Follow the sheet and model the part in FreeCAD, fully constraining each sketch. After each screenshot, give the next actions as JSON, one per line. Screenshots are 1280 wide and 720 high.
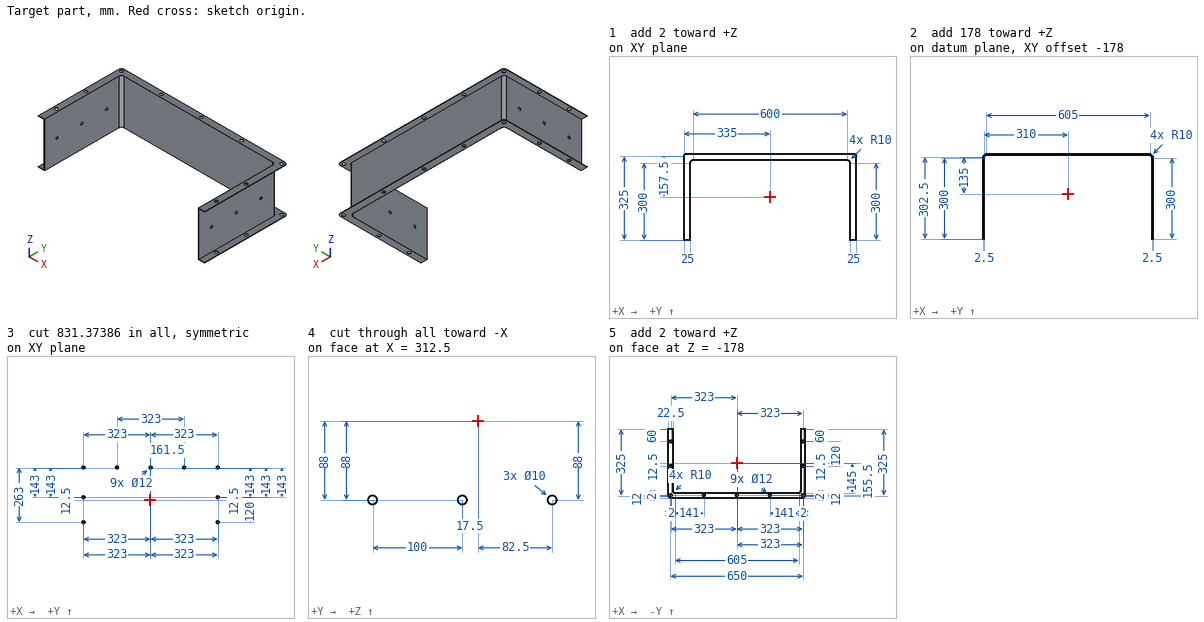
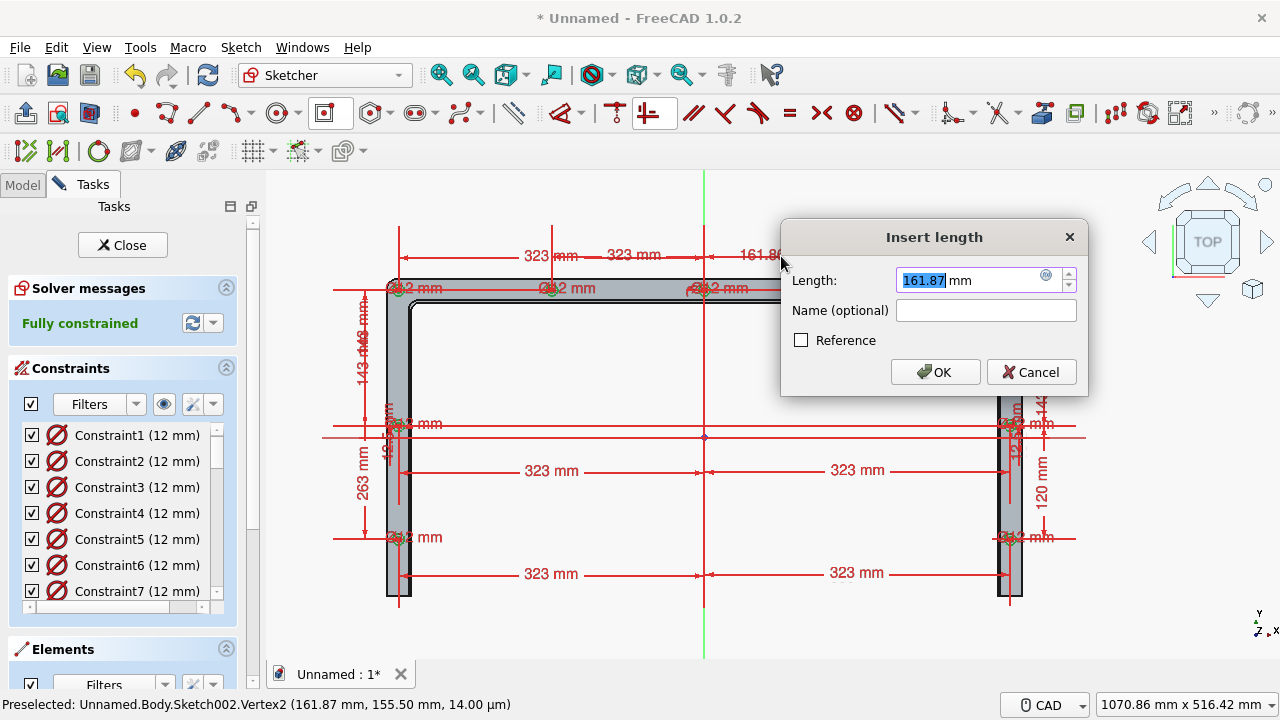
{"action": "type", "text": "161.5"}
{"action": "key", "text": "Return"}
{"action": "key", "text": "Escape"}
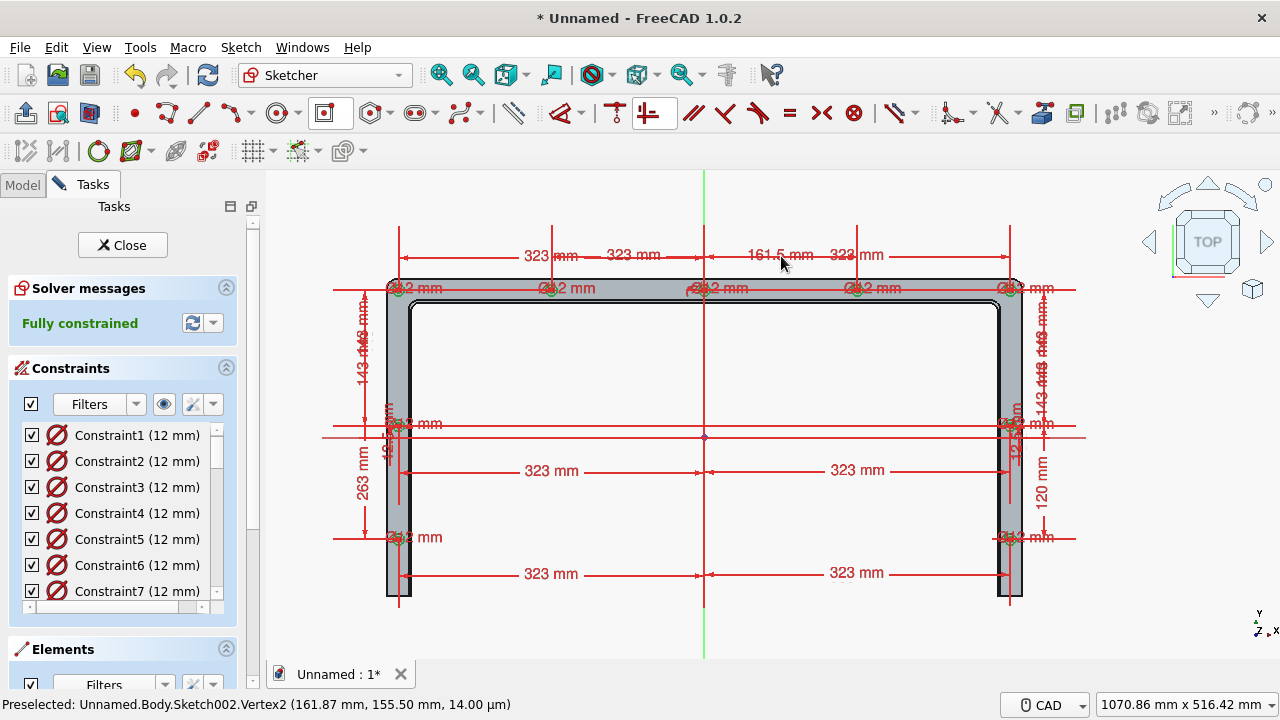
{"action": "left_click", "coordinate": [123, 245]}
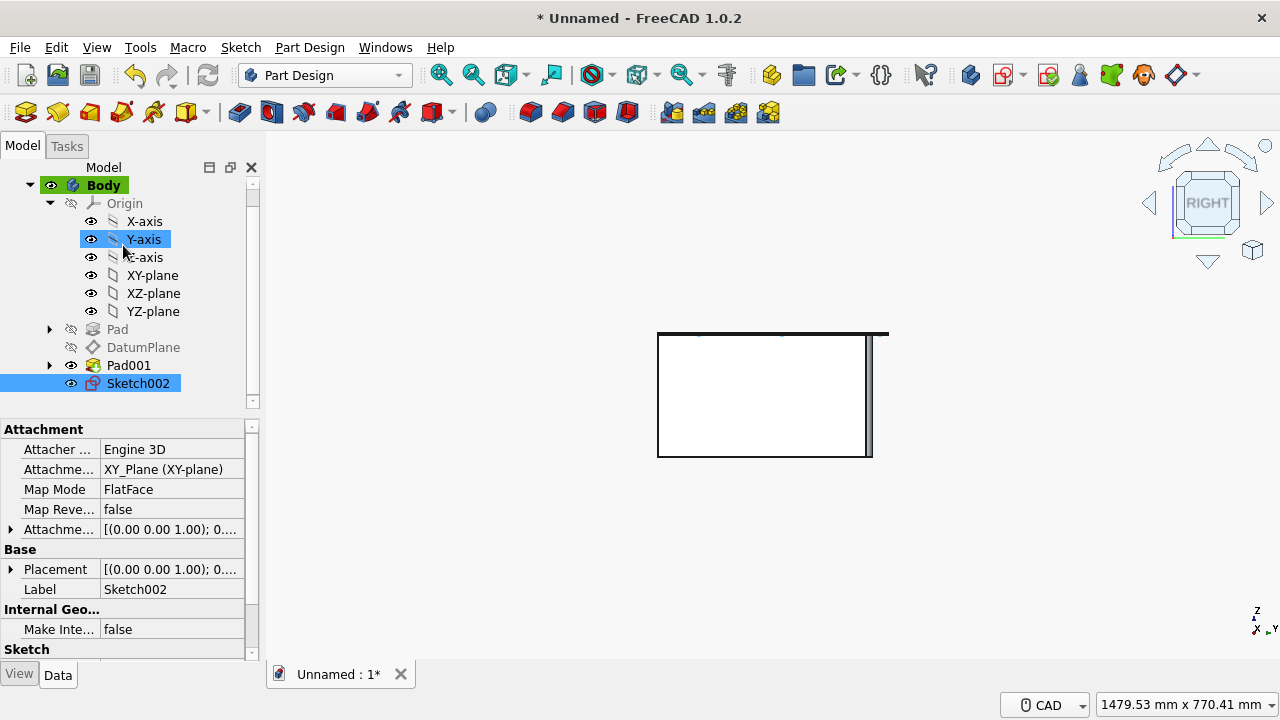
{"action": "left_click", "coordinate": [240, 112]}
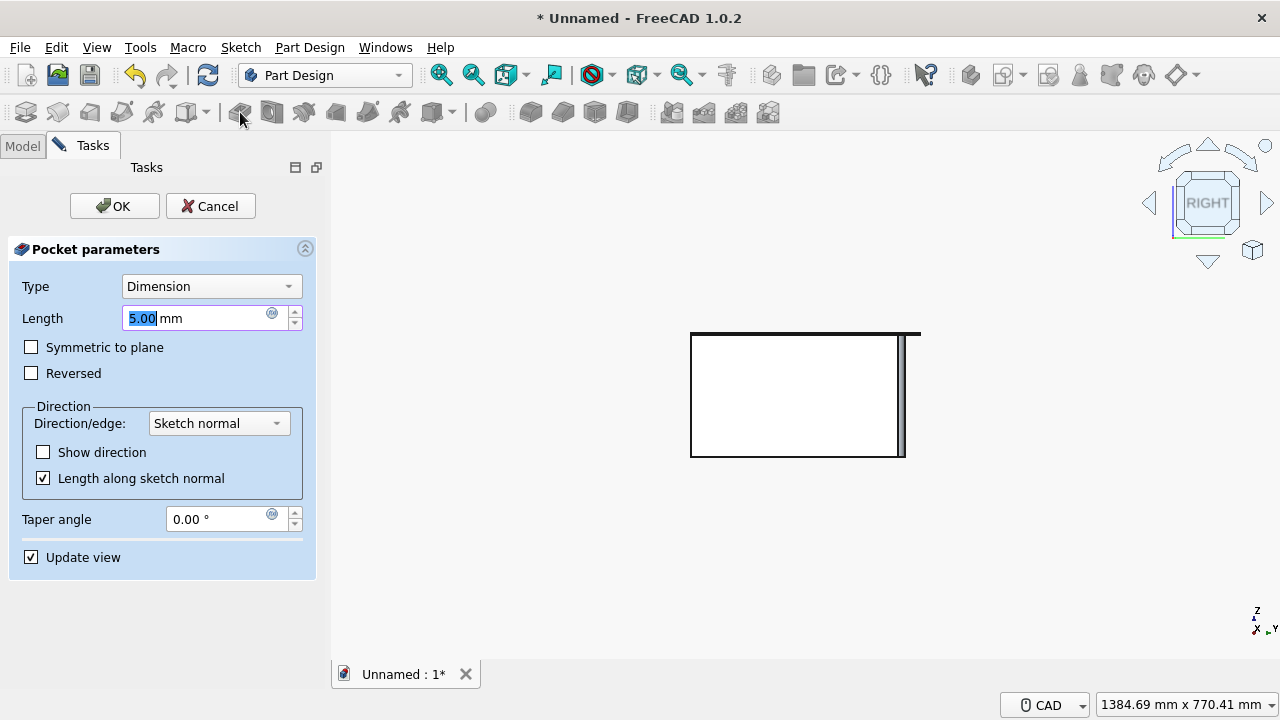
{"action": "type", "text": "831.37386"}
{"action": "key", "text": "Tab"}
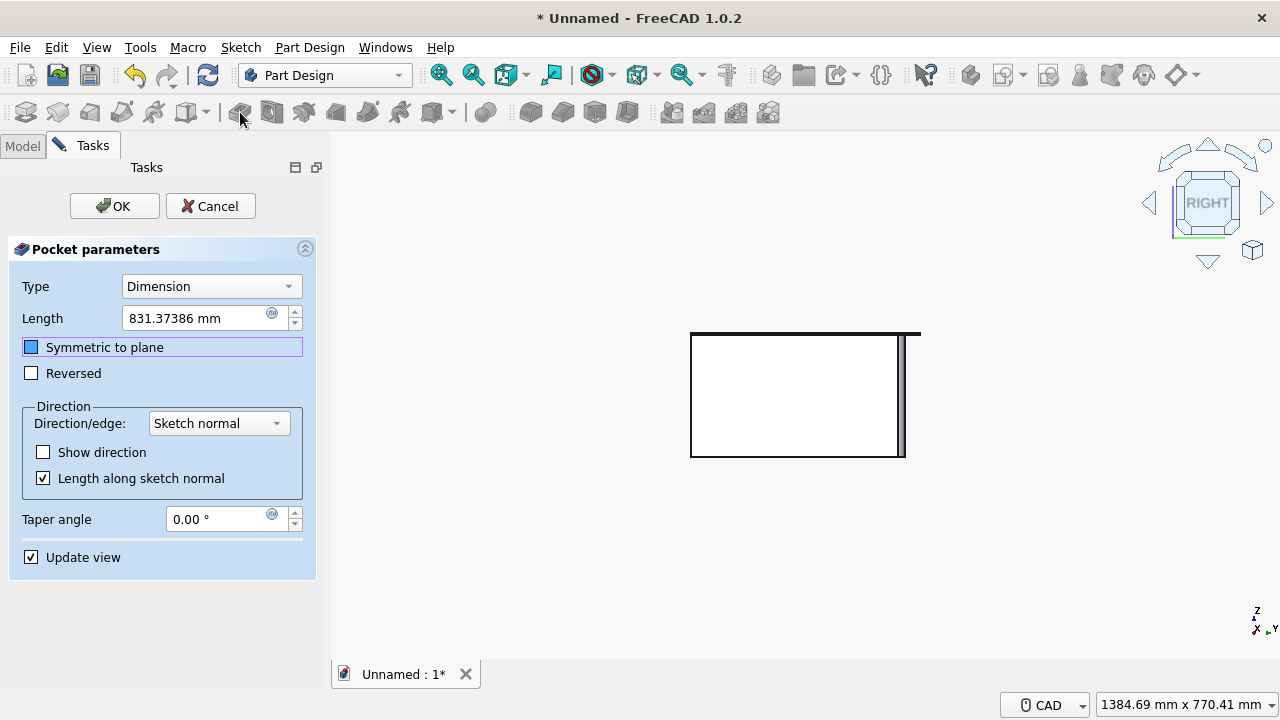
{"action": "left_click", "coordinate": [30, 347]}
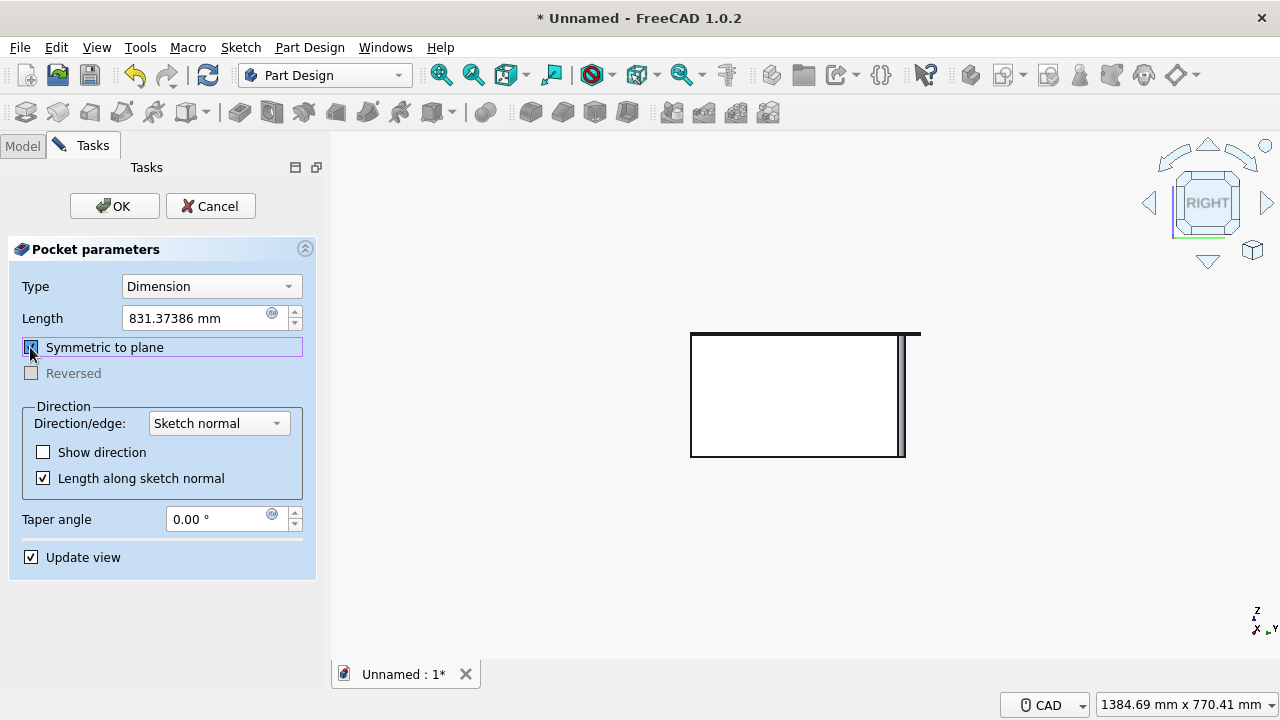
{"action": "left_click", "coordinate": [115, 206]}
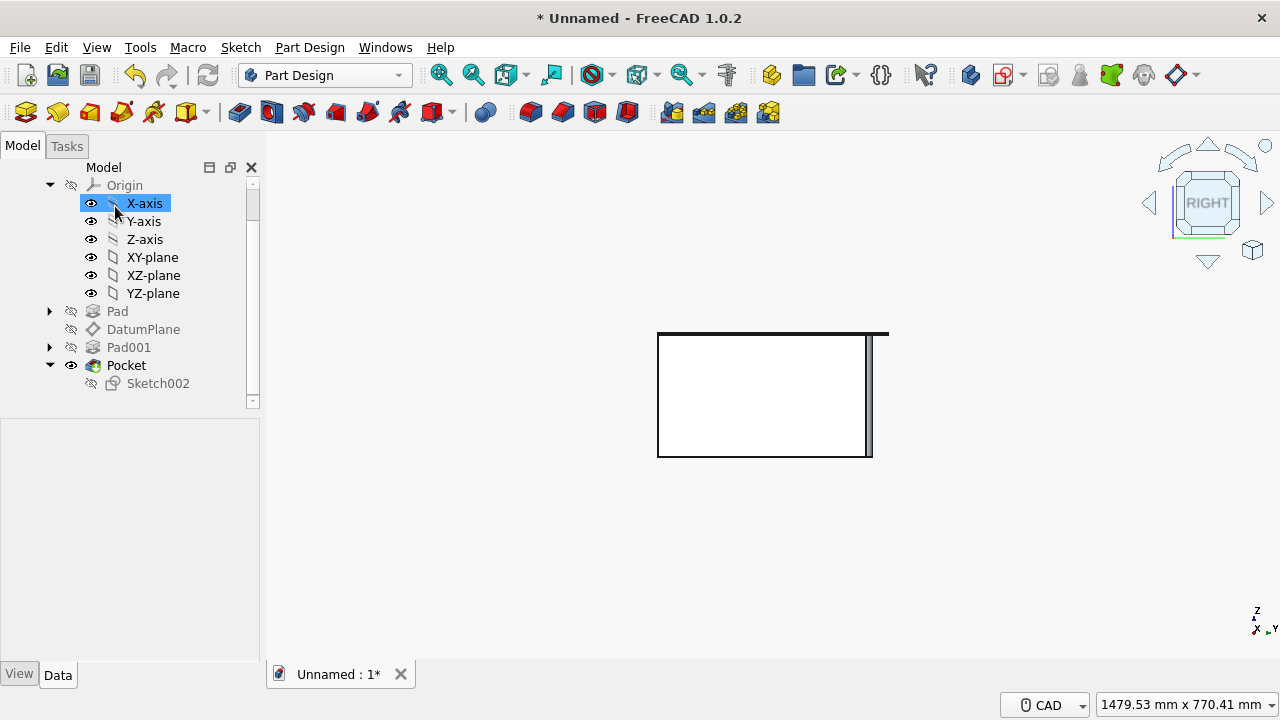
{"action": "left_click", "coordinate": [442, 76]}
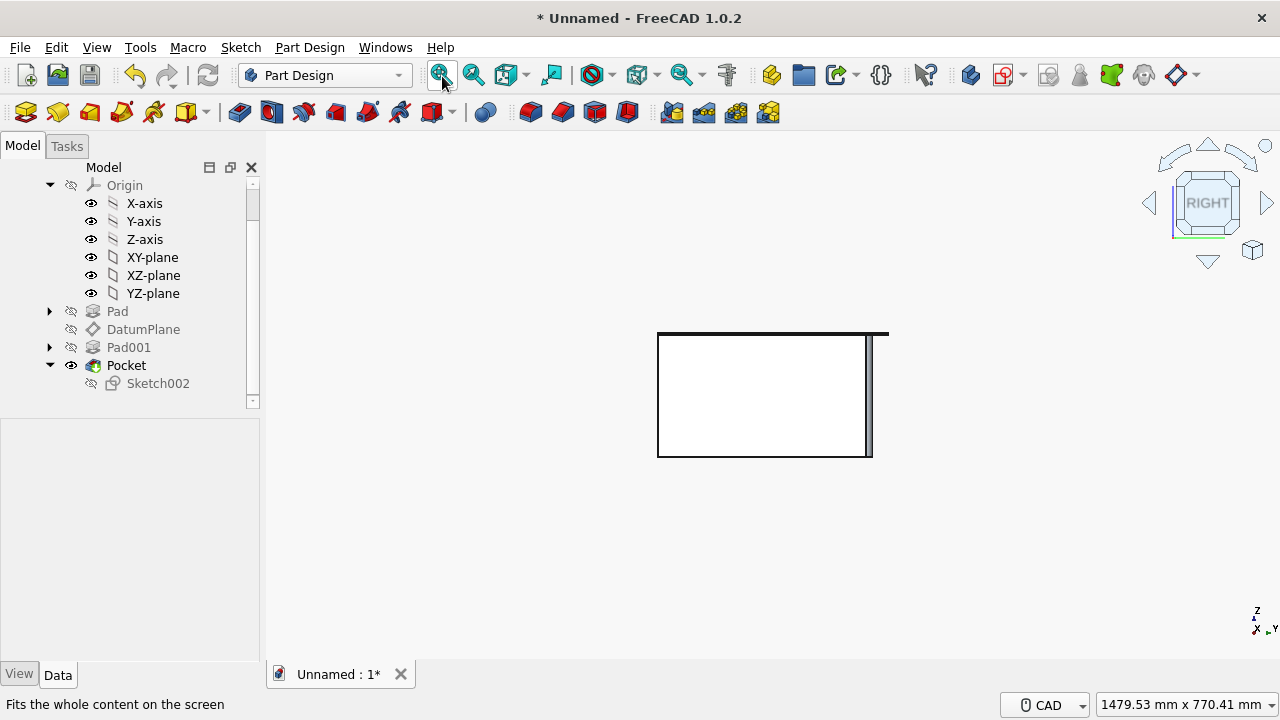
{"action": "left_click", "coordinate": [791, 395]}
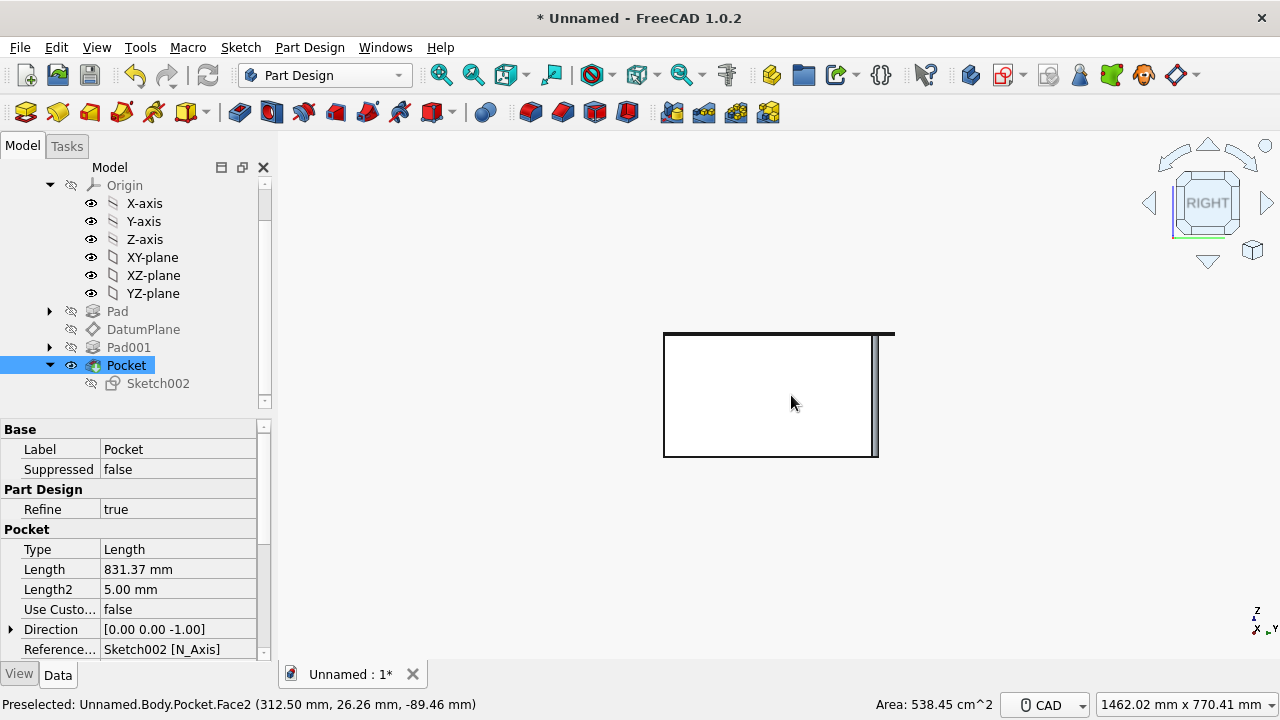
{"action": "left_click", "coordinate": [1004, 76]}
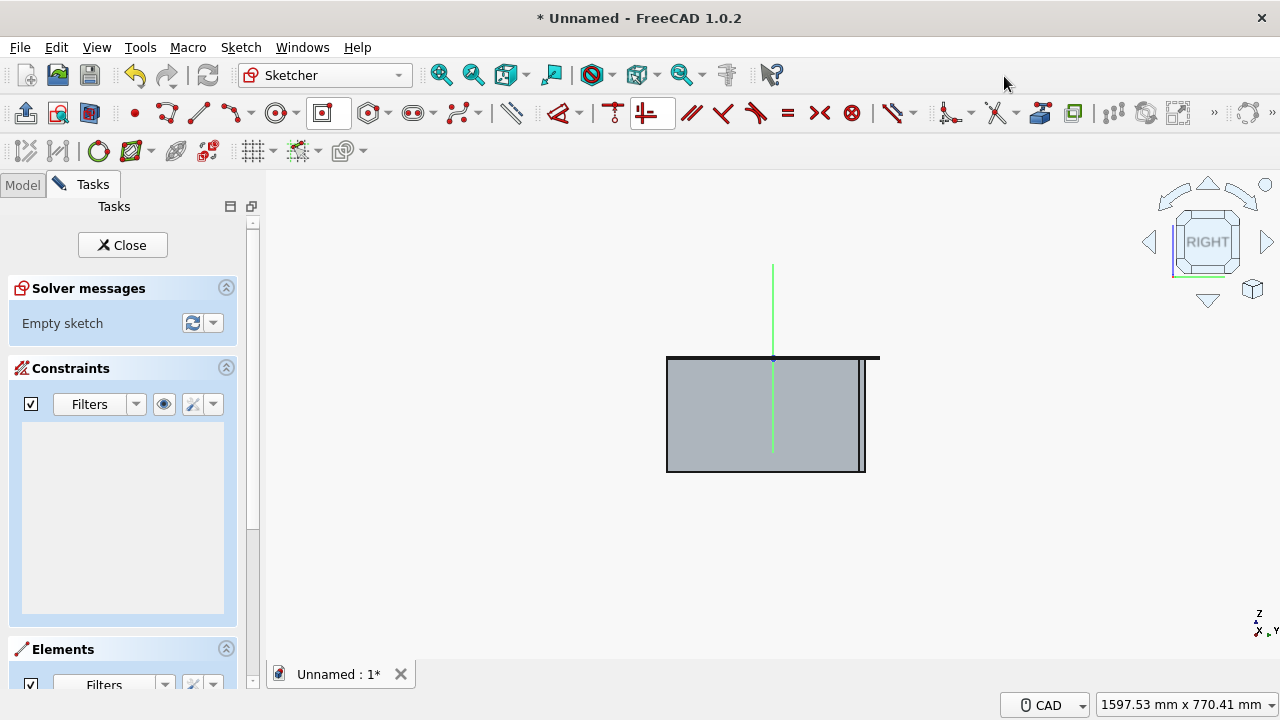
{"action": "scroll", "coordinate": [781, 380], "scroll_direction": "up", "scroll_amount": 7}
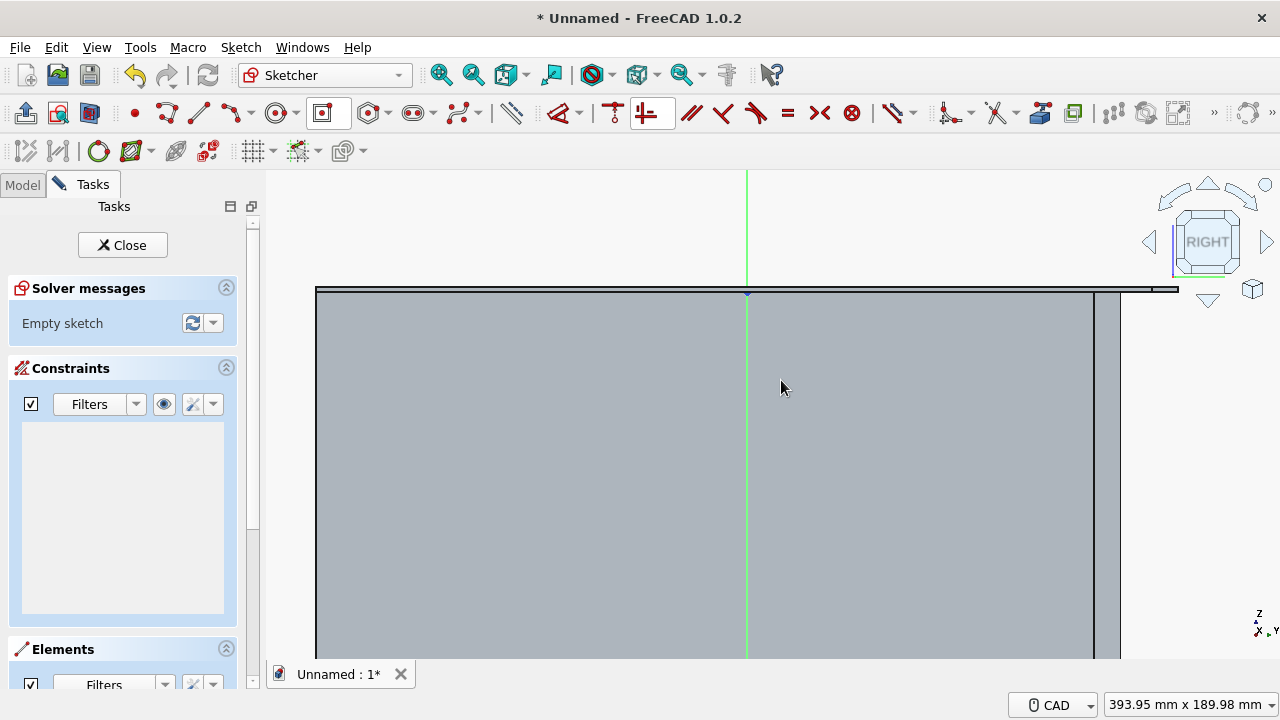
{"action": "left_click", "coordinate": [276, 114]}